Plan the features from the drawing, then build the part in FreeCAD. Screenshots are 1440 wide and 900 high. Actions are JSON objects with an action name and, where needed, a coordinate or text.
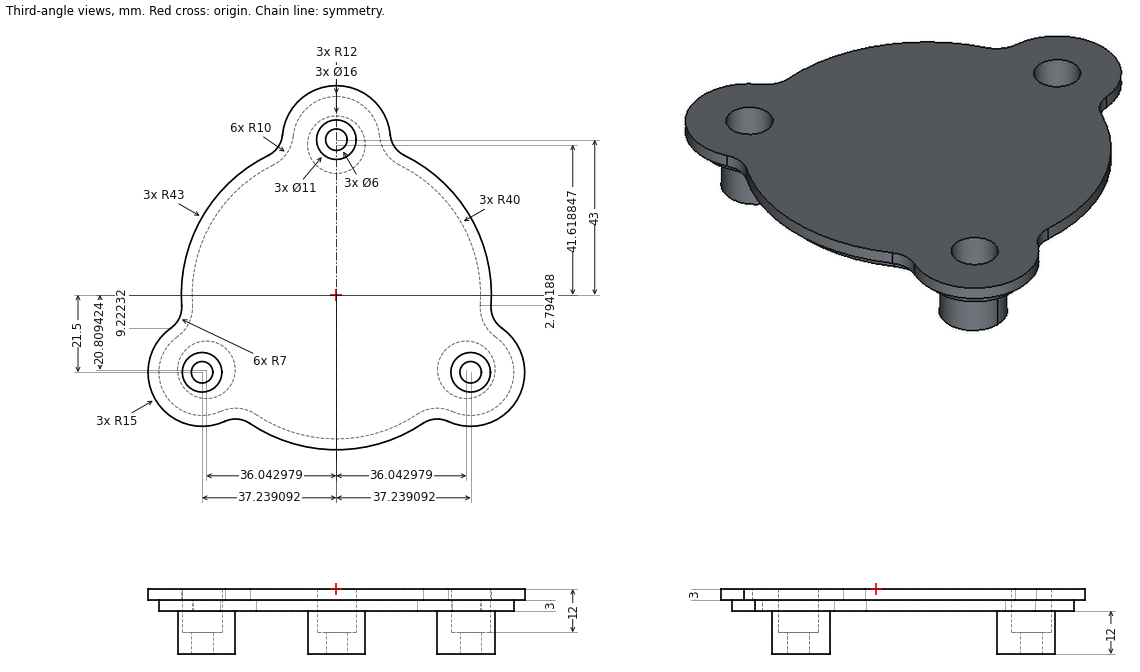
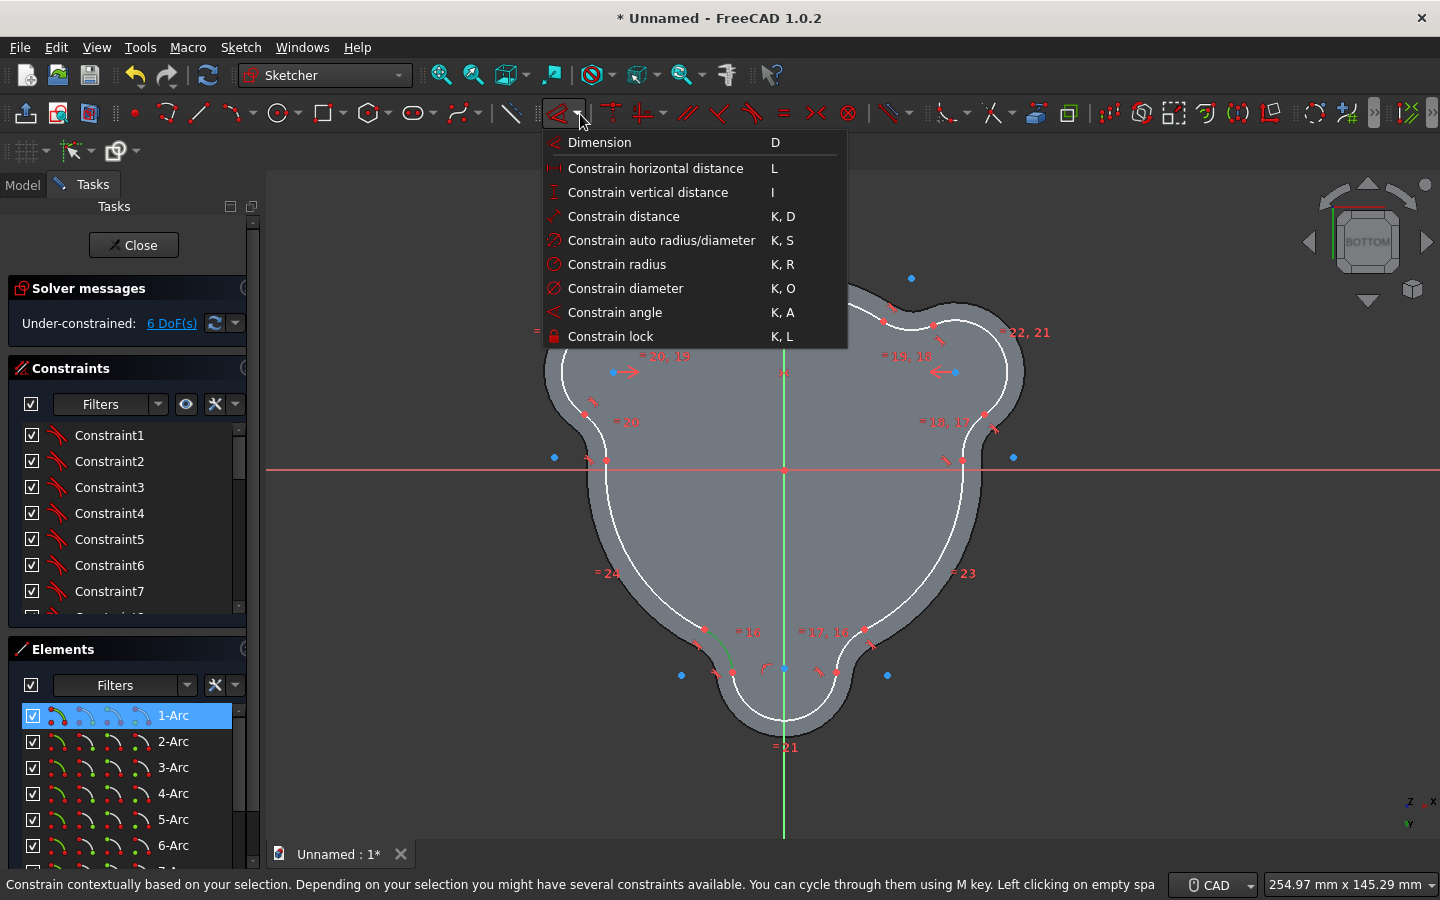
{"action": "left_click", "coordinate": [695, 264]}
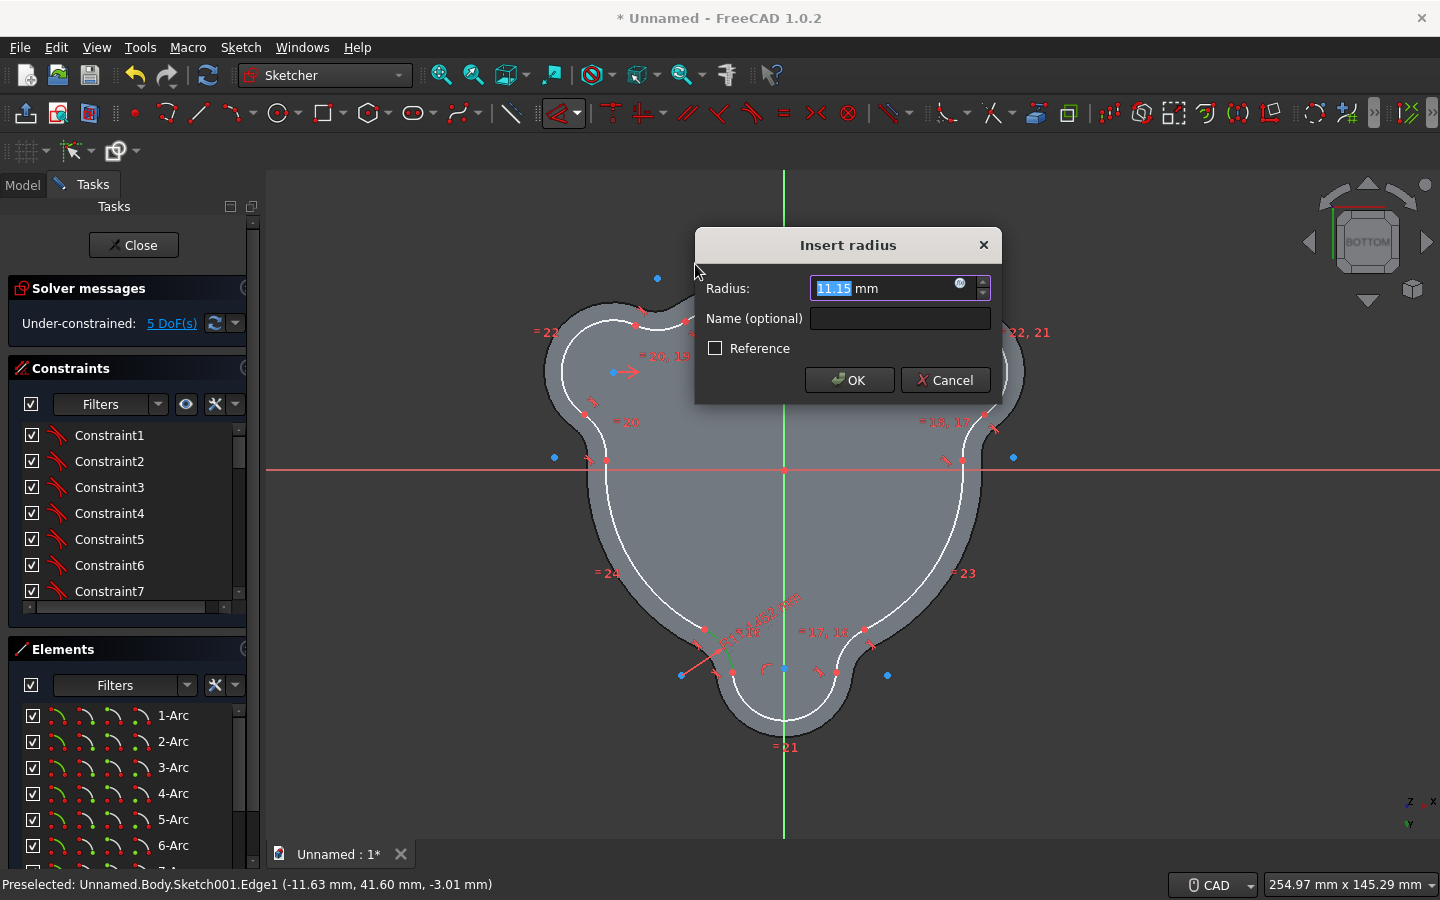
{"action": "type", "text": "10"}
{"action": "key", "text": "Return"}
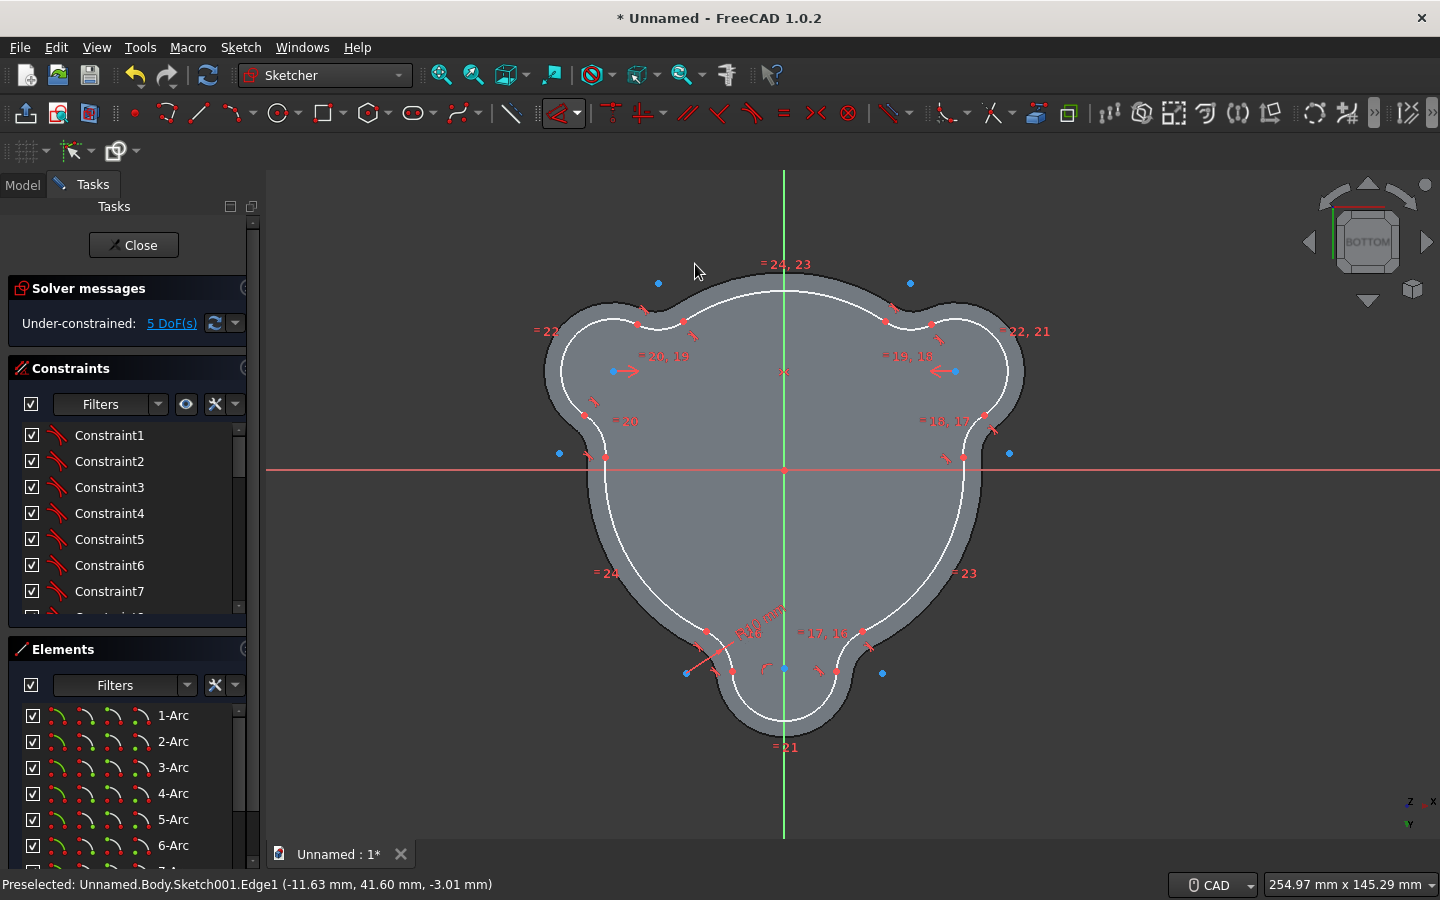
{"action": "left_click", "coordinate": [754, 712]}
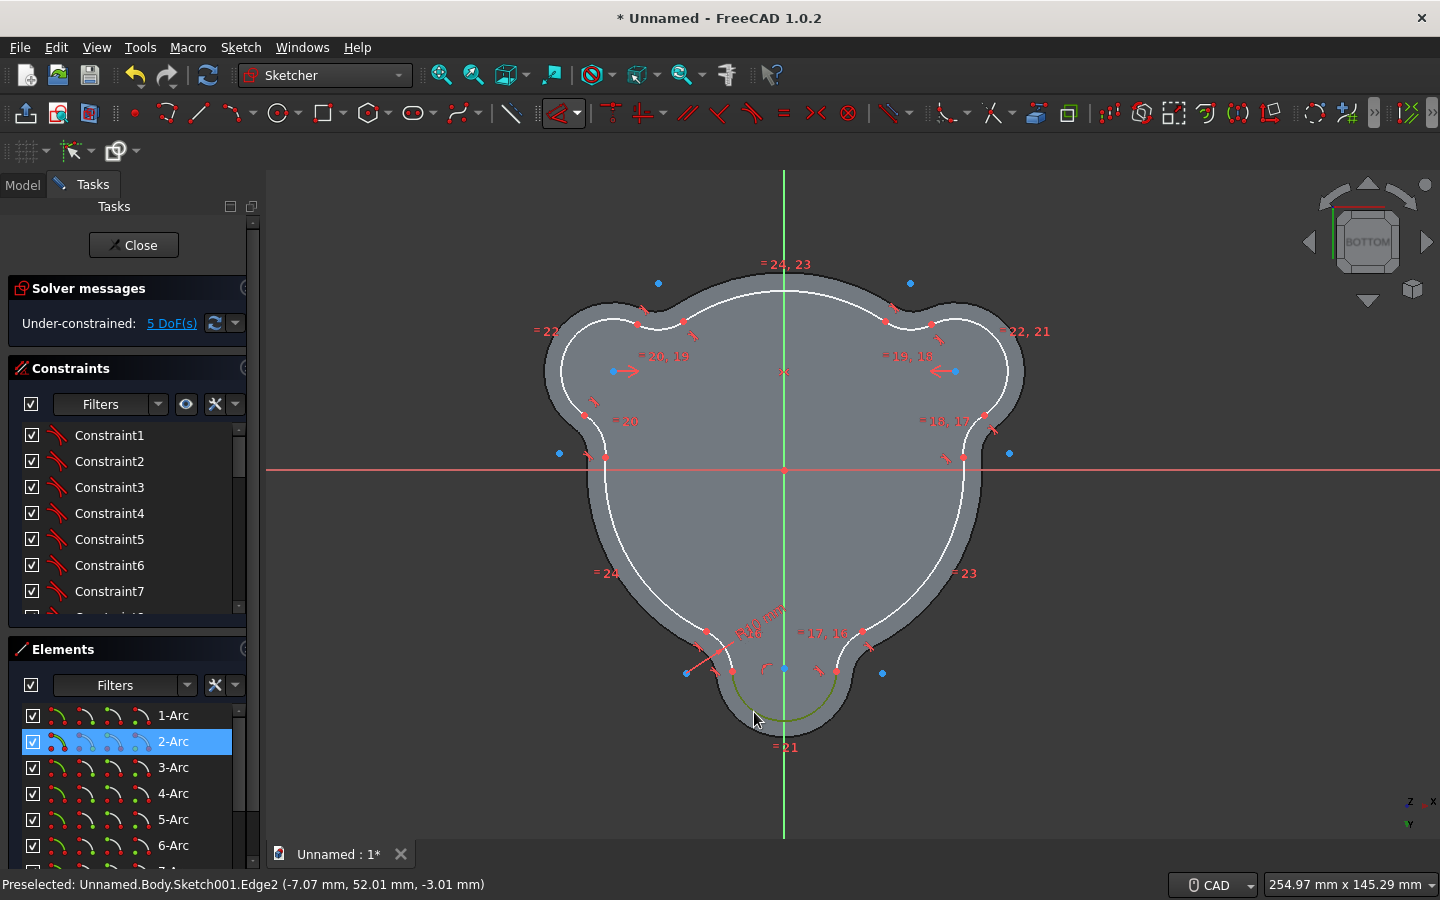
{"action": "left_click", "coordinate": [580, 114]}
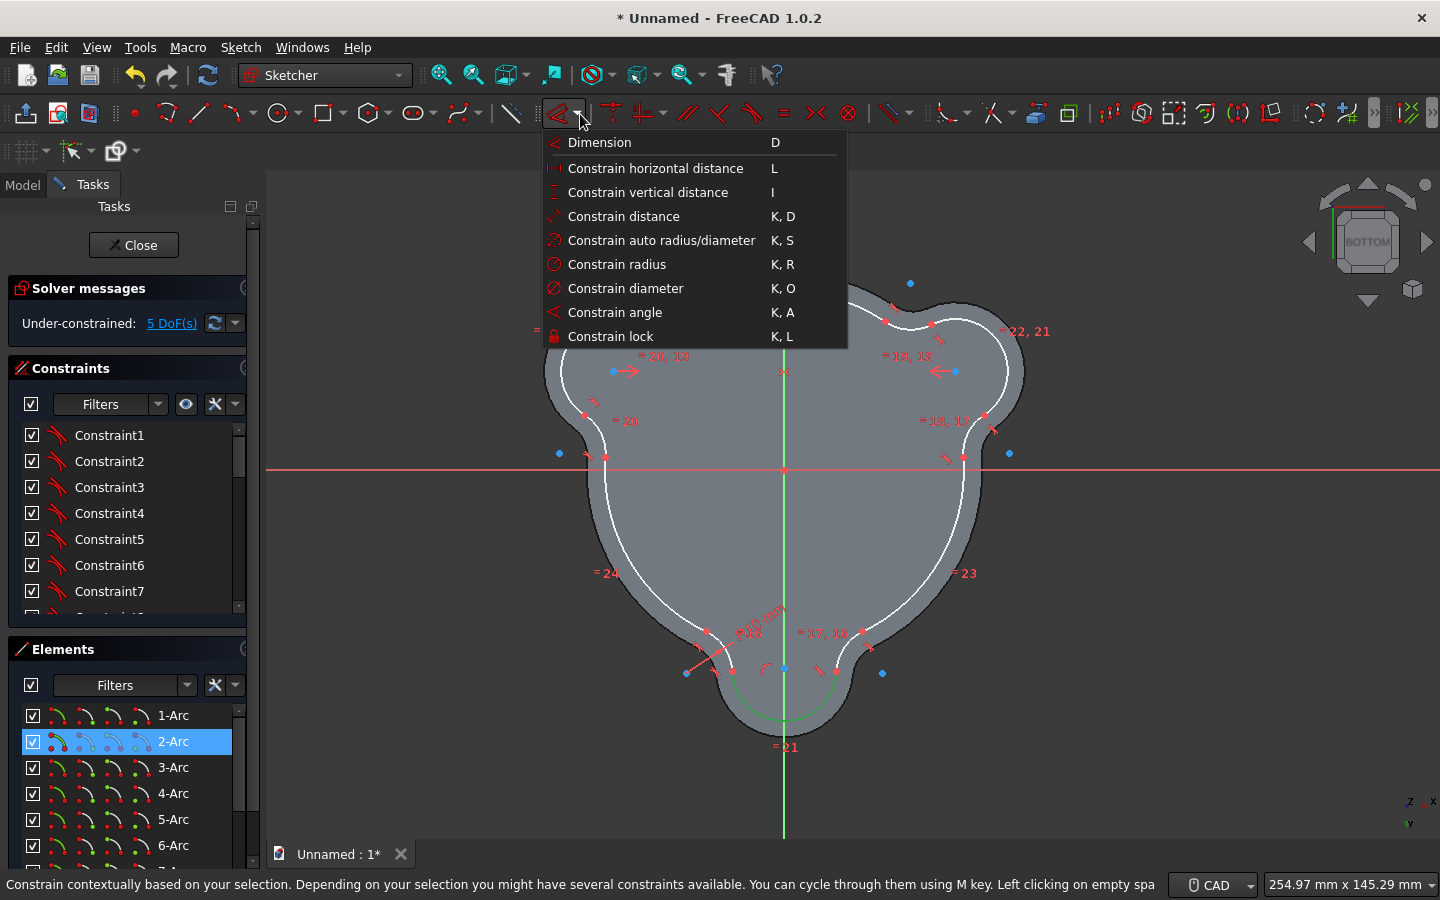
{"action": "left_click", "coordinate": [695, 264]}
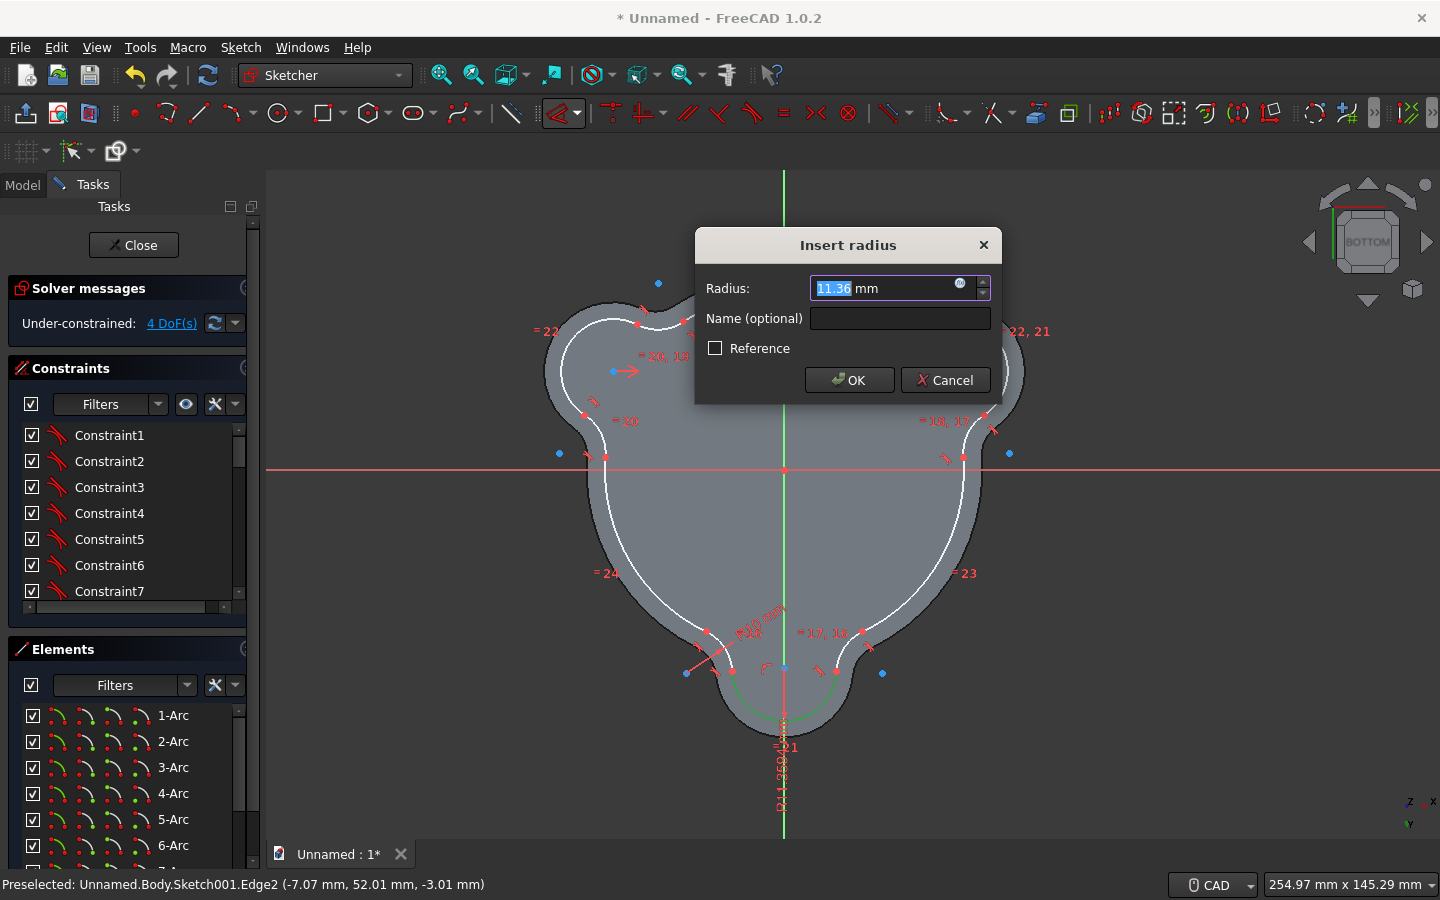
{"action": "type", "text": "12"}
{"action": "key", "text": "Return"}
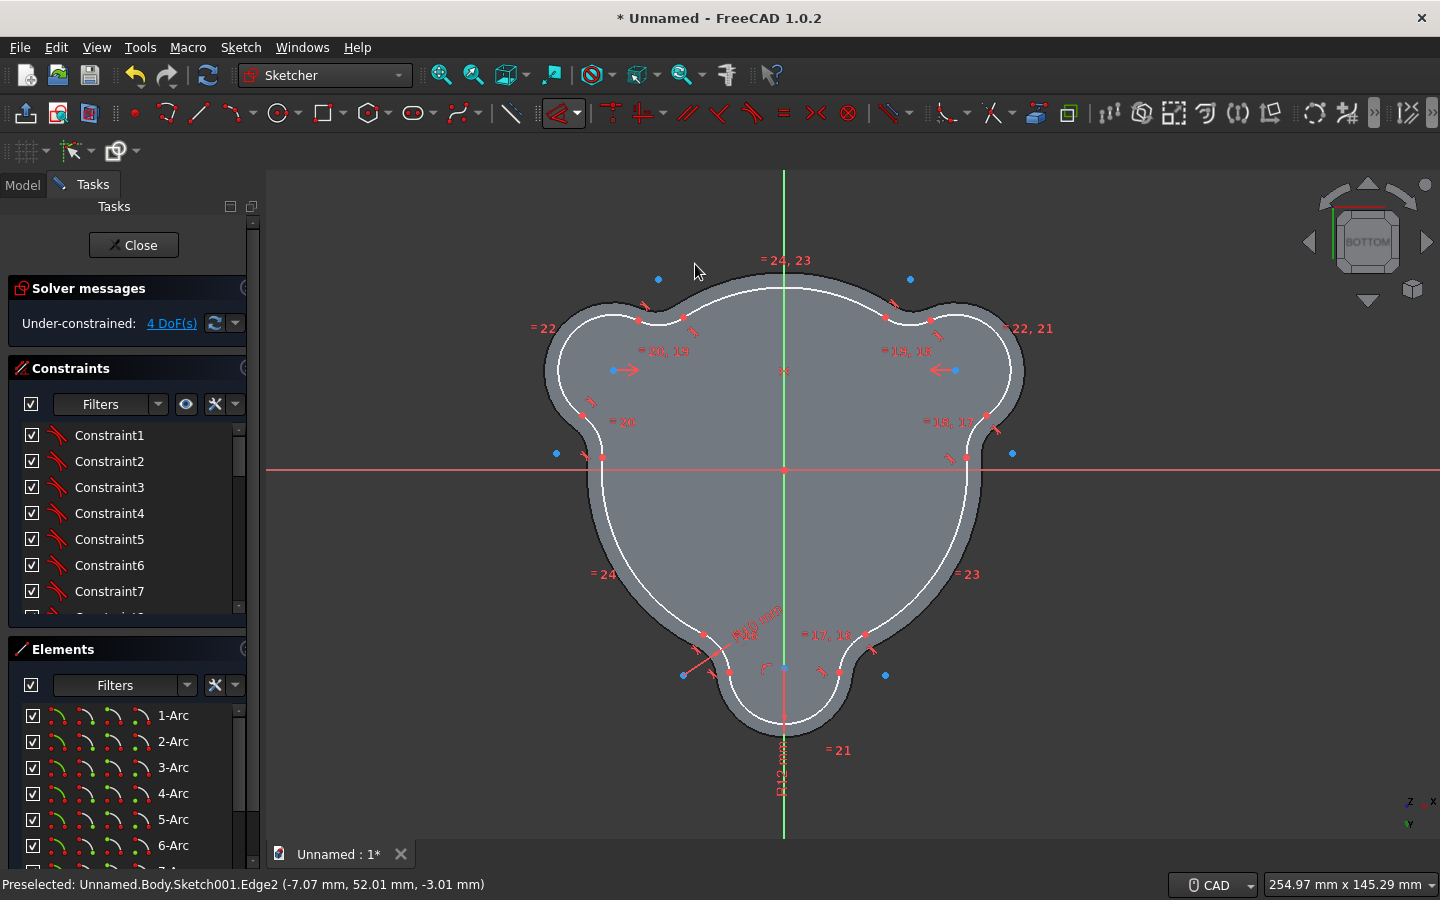
{"action": "left_click", "coordinate": [917, 596]}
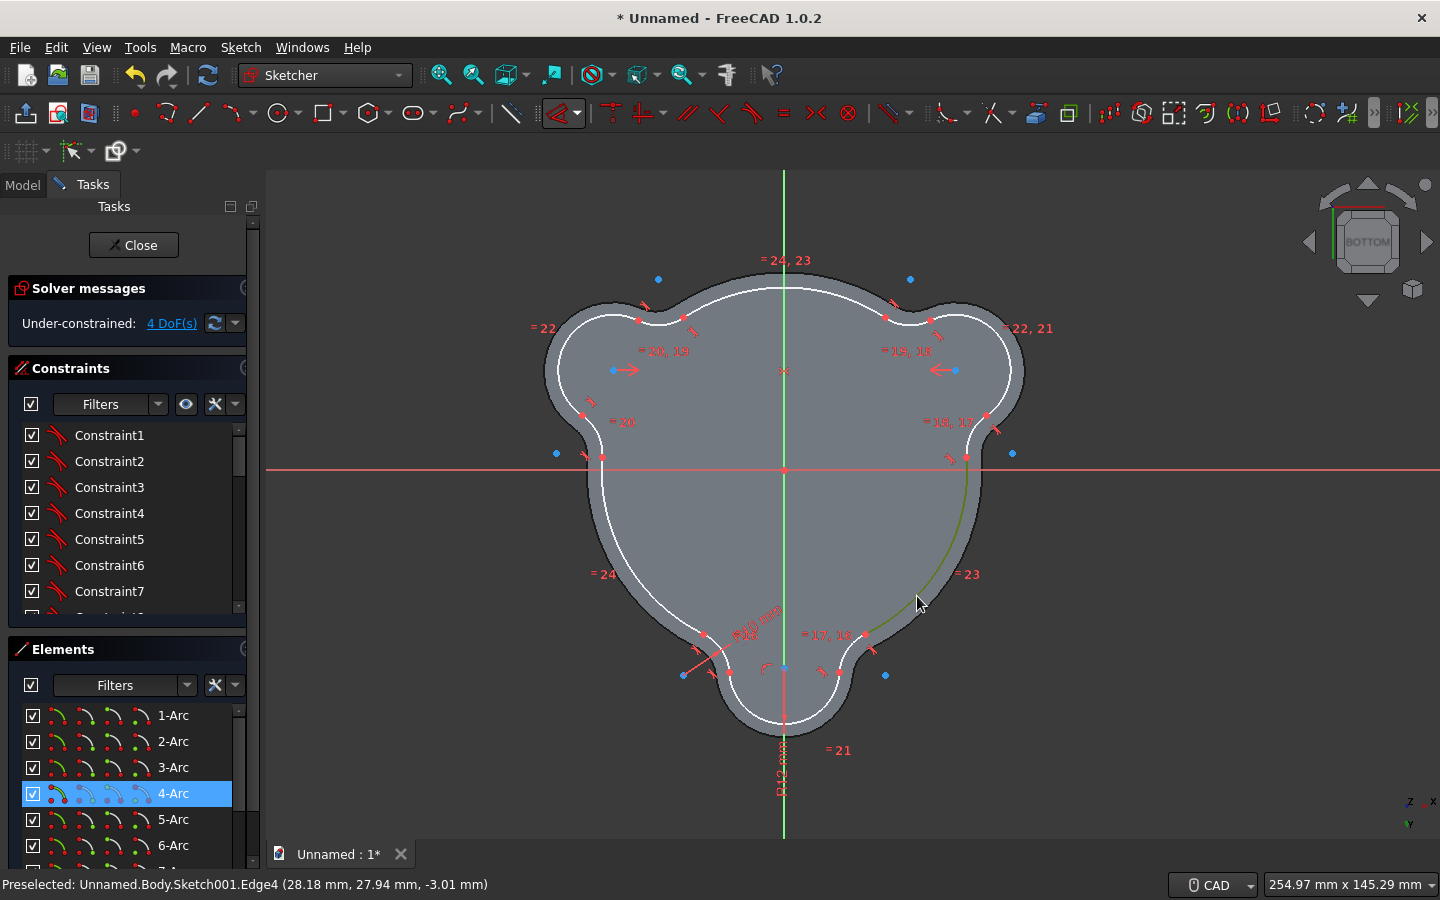
{"action": "key", "text": "k r"}